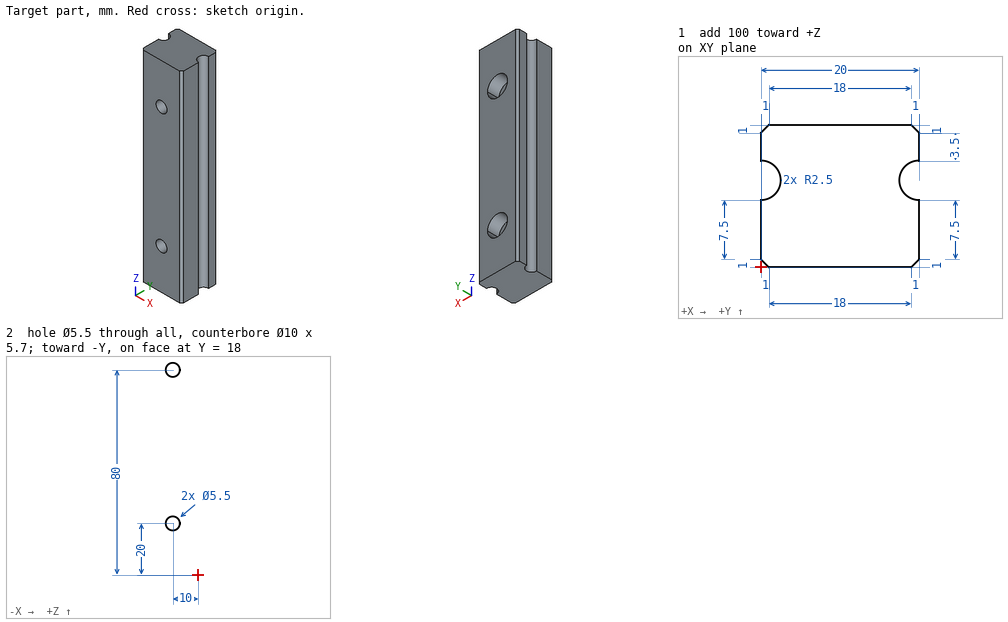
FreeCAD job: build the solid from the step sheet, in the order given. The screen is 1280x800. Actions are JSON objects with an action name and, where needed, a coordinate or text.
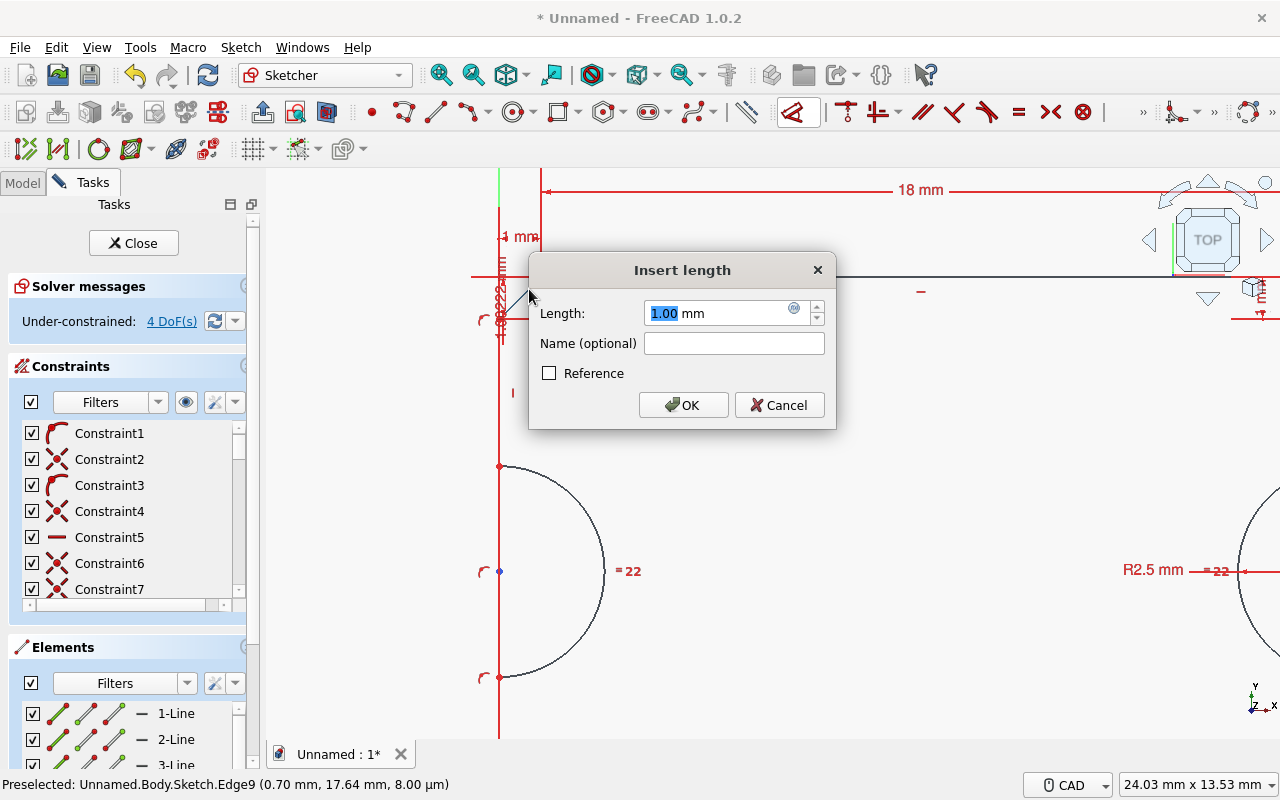
{"action": "type", "text": "1"}
{"action": "key", "text": "Return"}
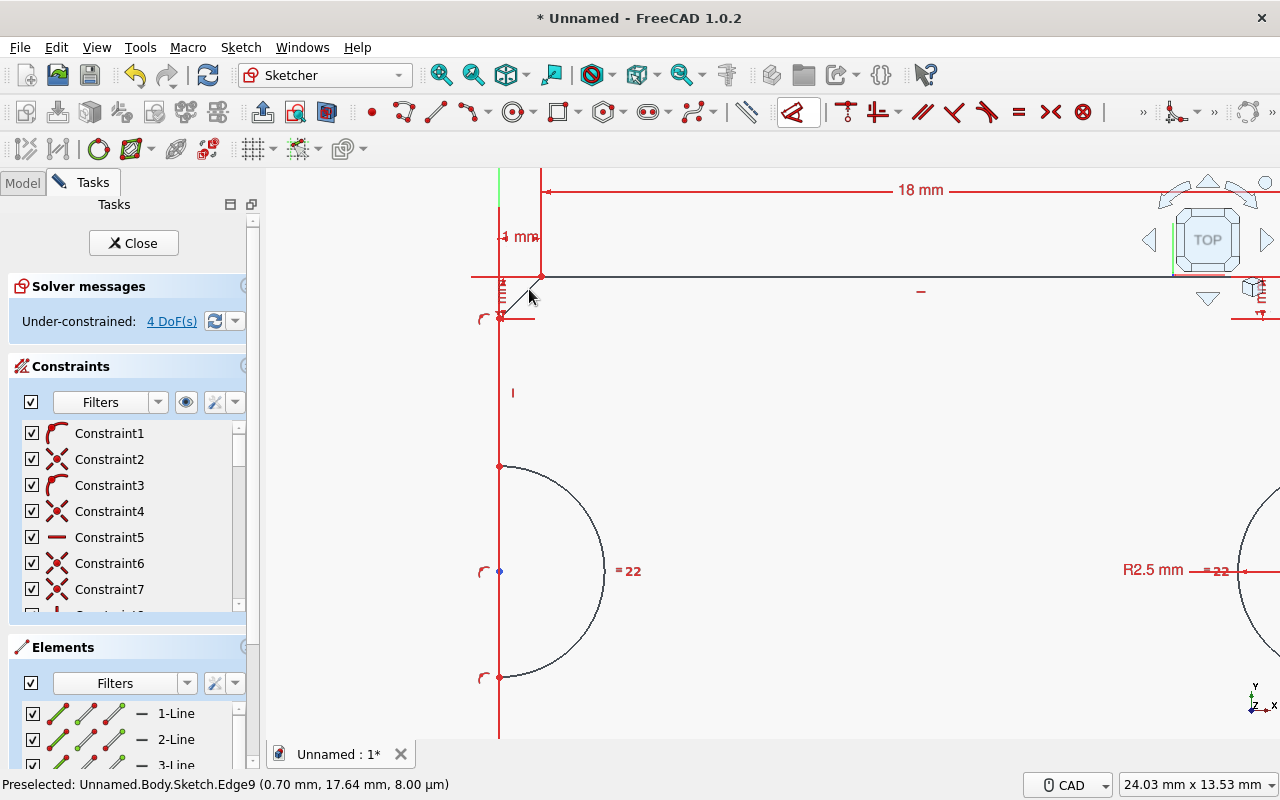
{"action": "scroll", "coordinate": [528, 290], "scroll_direction": "down", "scroll_amount": 4}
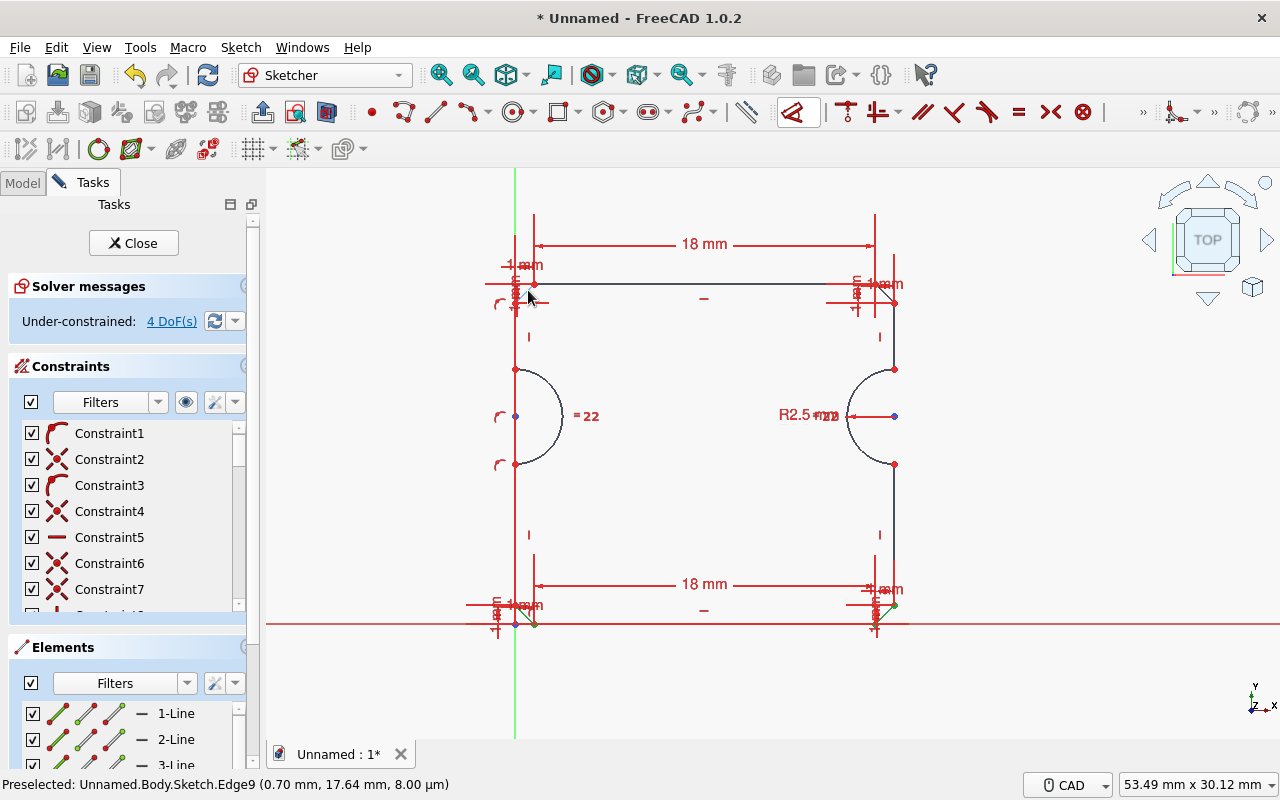
{"action": "left_click", "coordinate": [515, 506]}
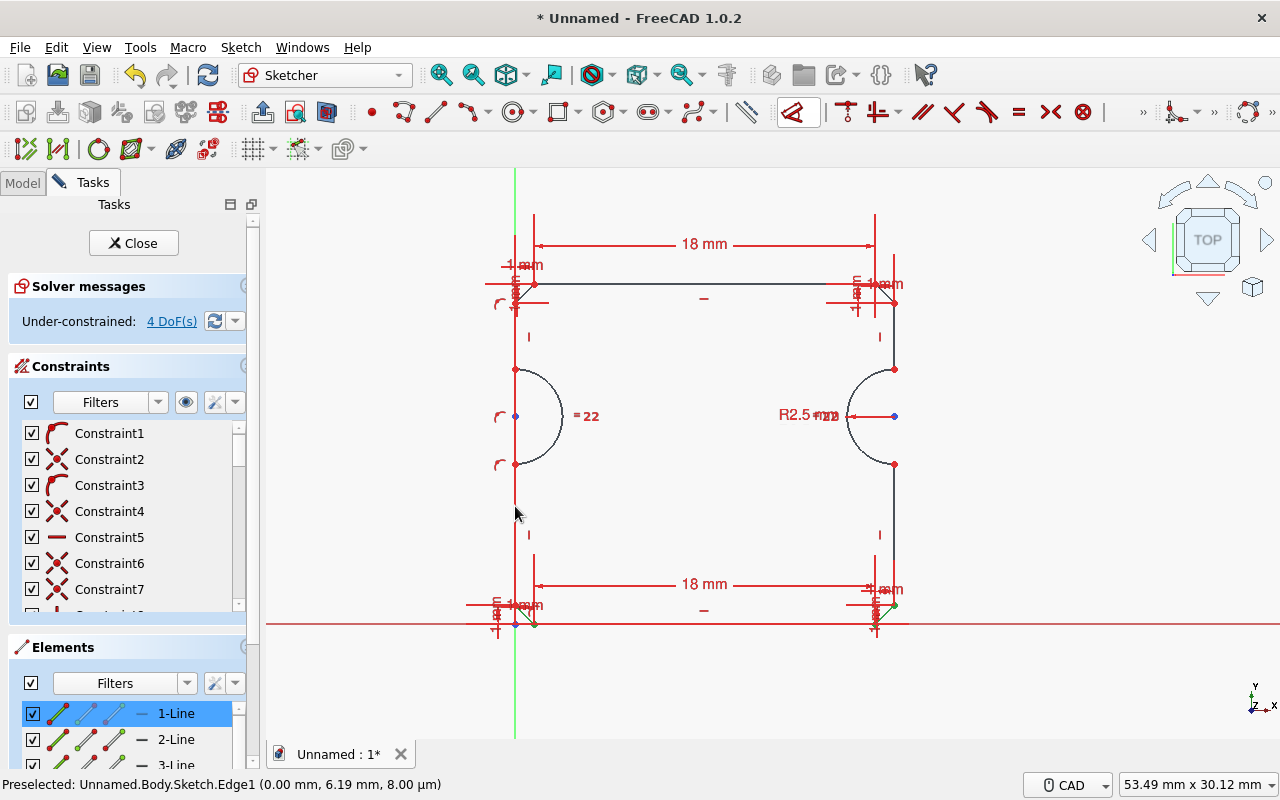
{"action": "left_click", "coordinate": [814, 112]}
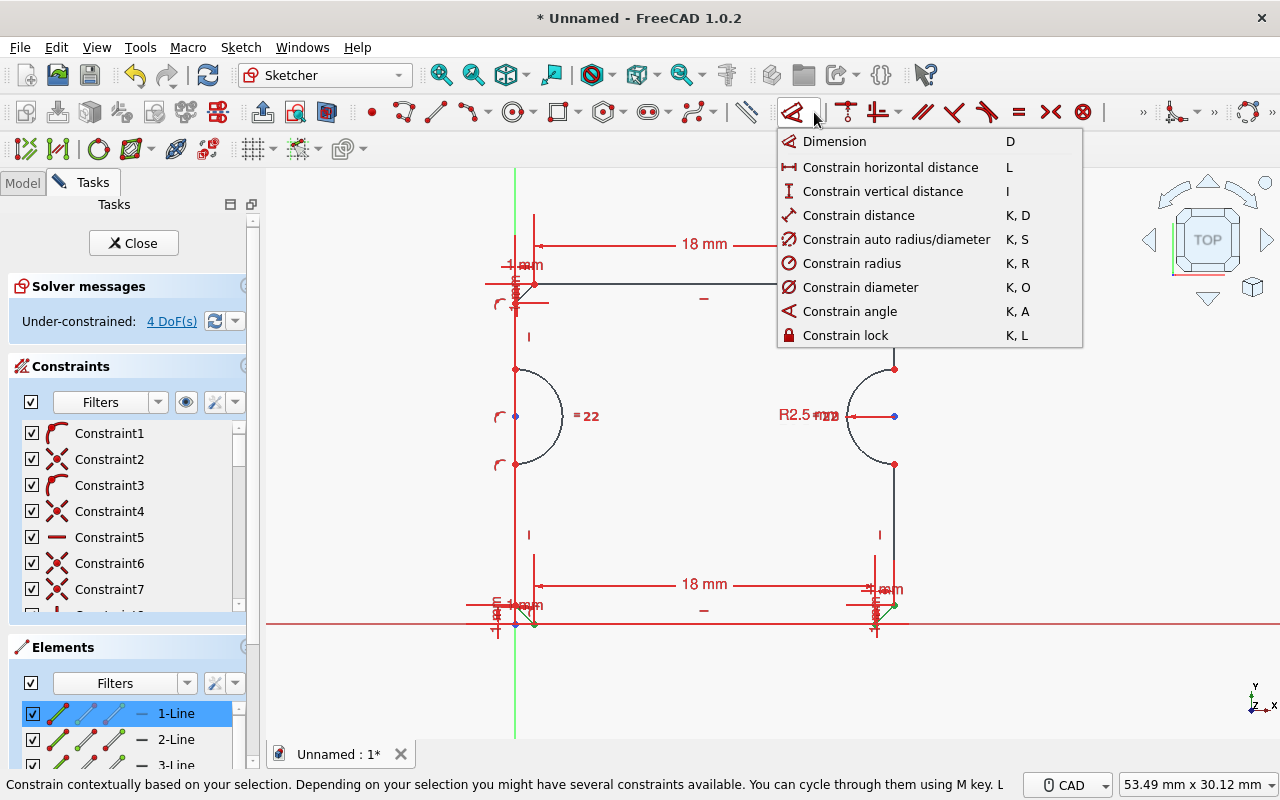
{"action": "left_click", "coordinate": [930, 191]}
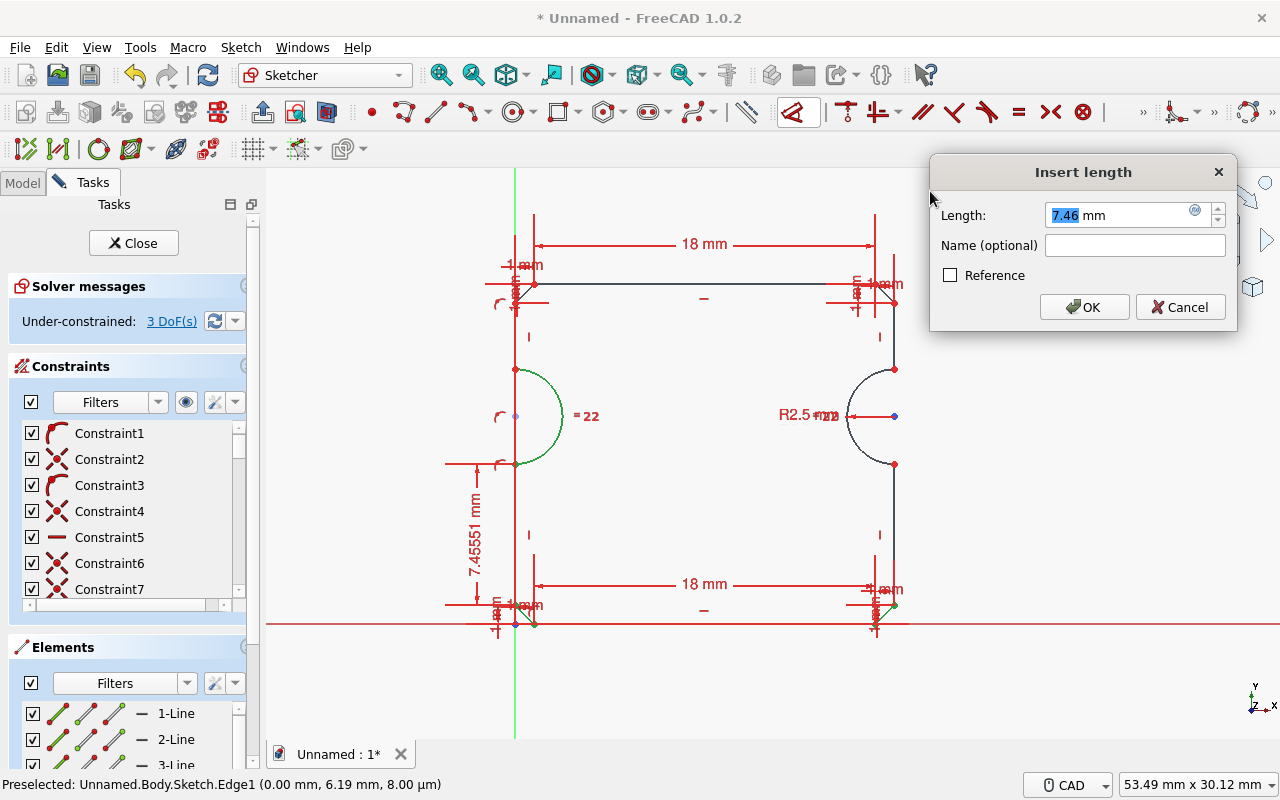
{"action": "type", "text": "7.5"}
{"action": "key", "text": "Return"}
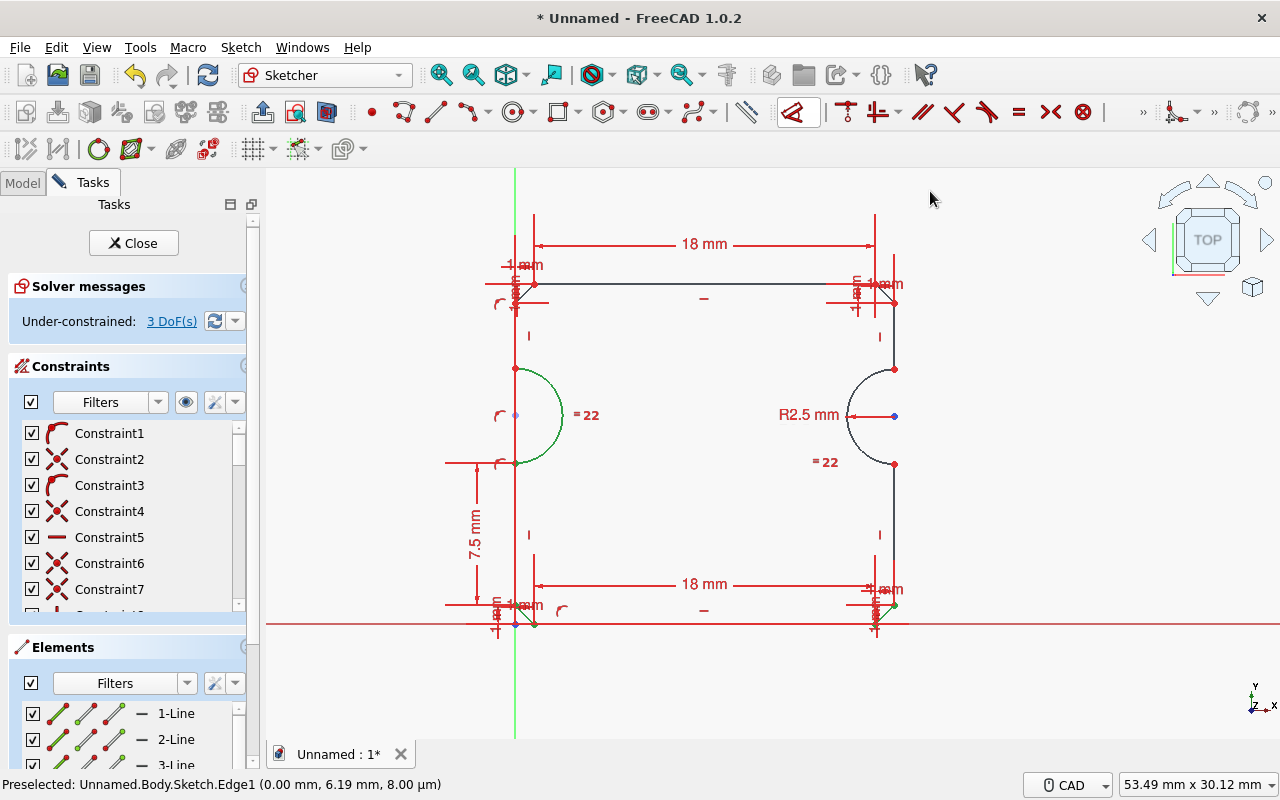
{"action": "left_click", "coordinate": [894, 563]}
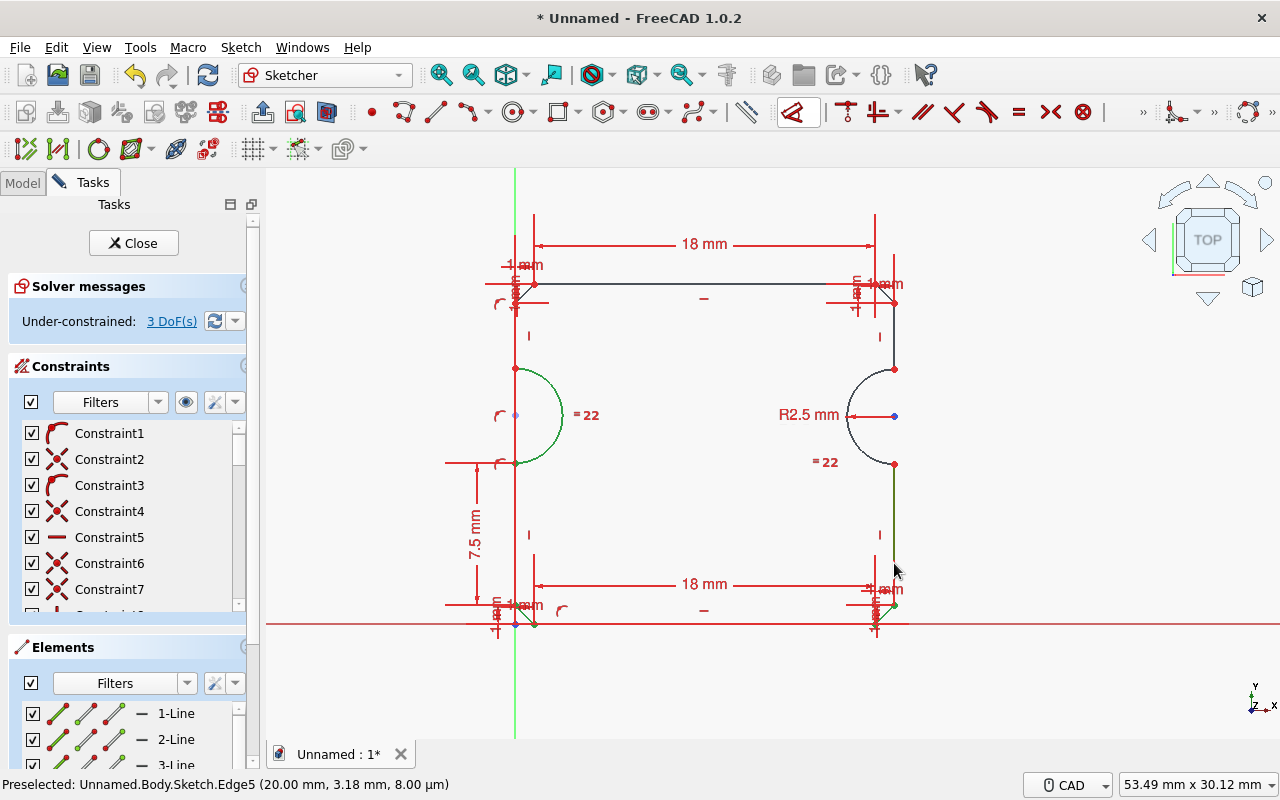
{"action": "left_click", "coordinate": [814, 112]}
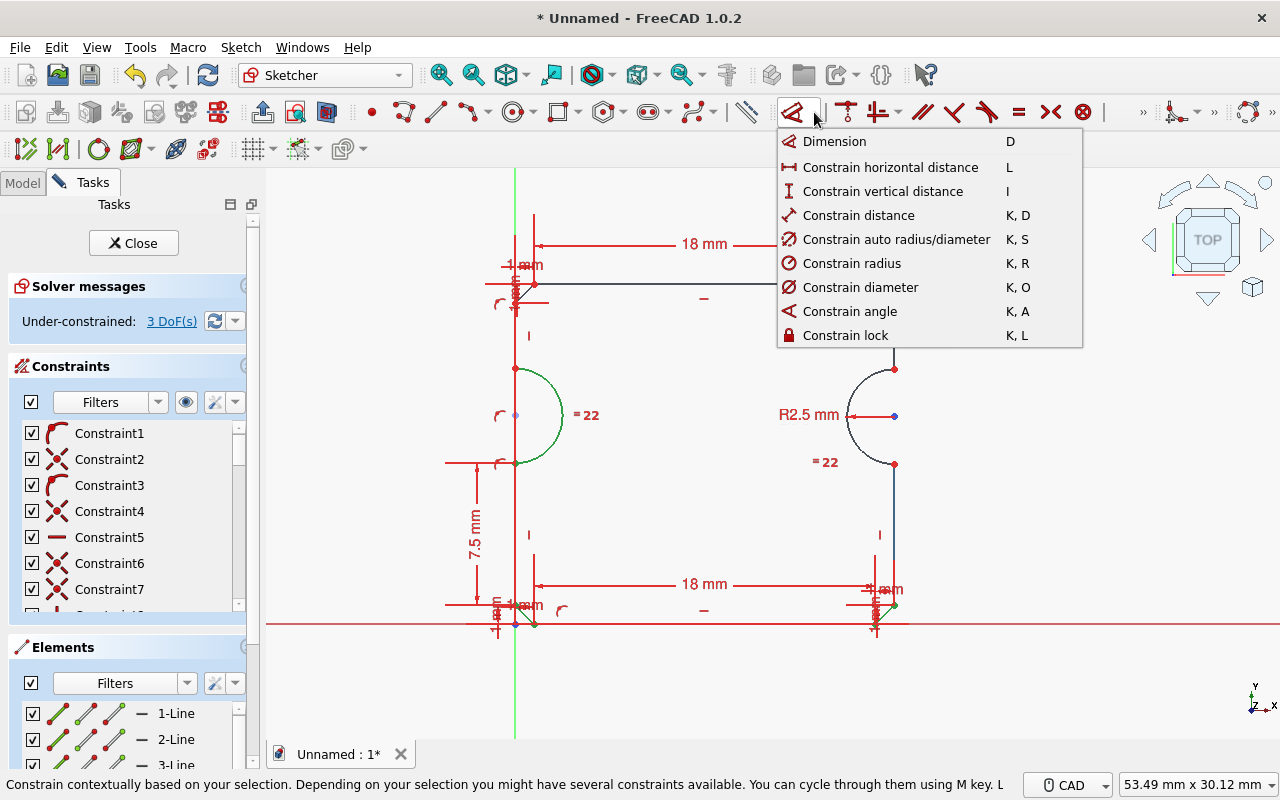
{"action": "left_click", "coordinate": [930, 191]}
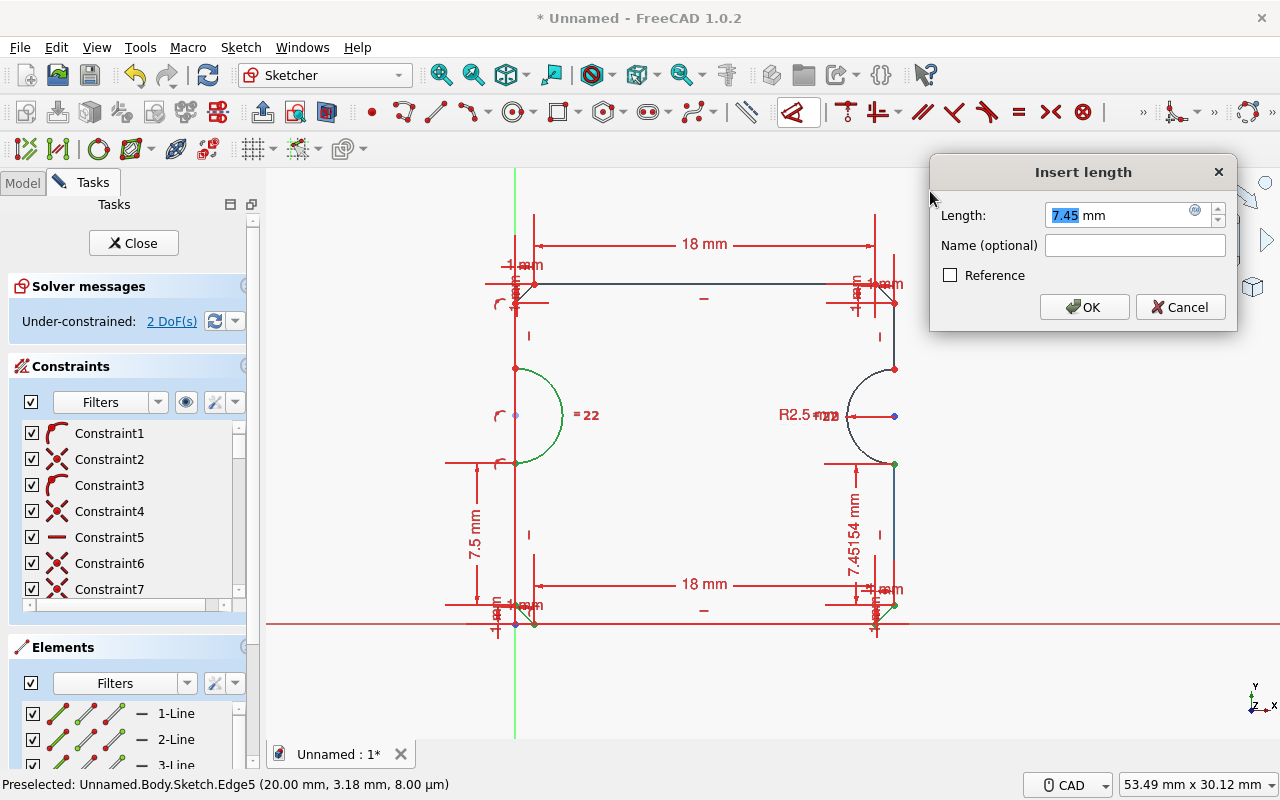
{"action": "type", "text": "7.5"}
{"action": "key", "text": "Return"}